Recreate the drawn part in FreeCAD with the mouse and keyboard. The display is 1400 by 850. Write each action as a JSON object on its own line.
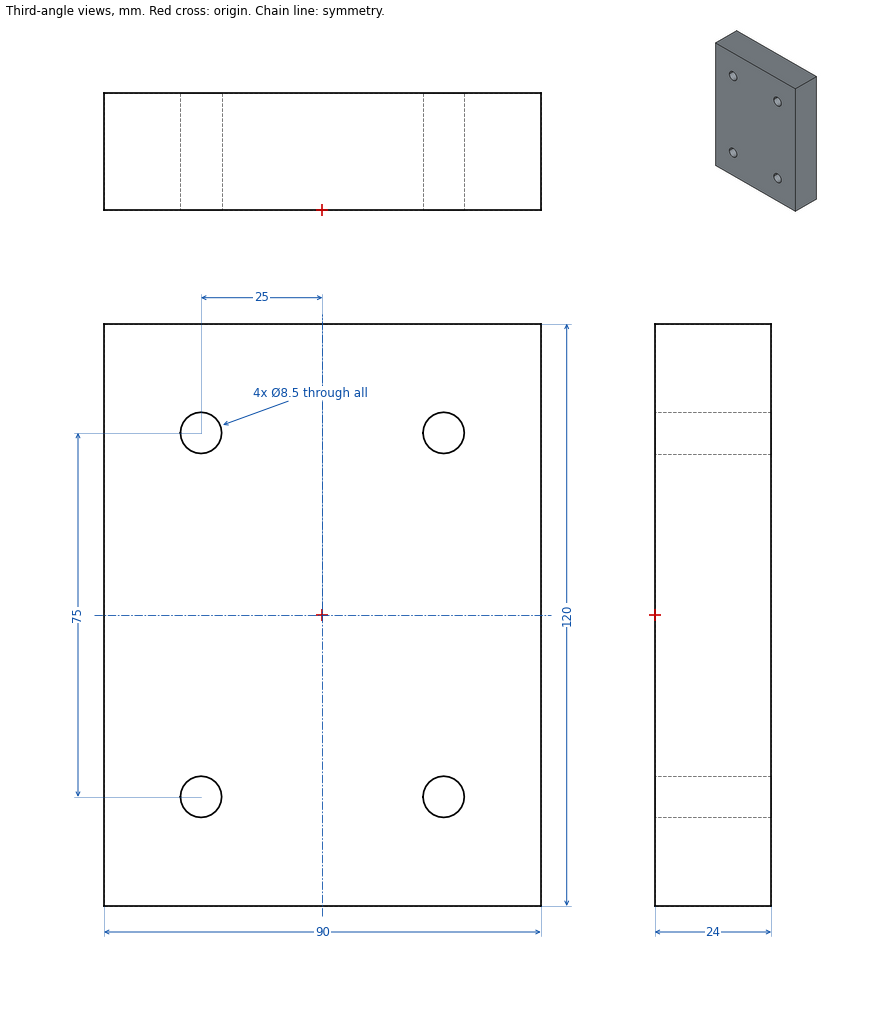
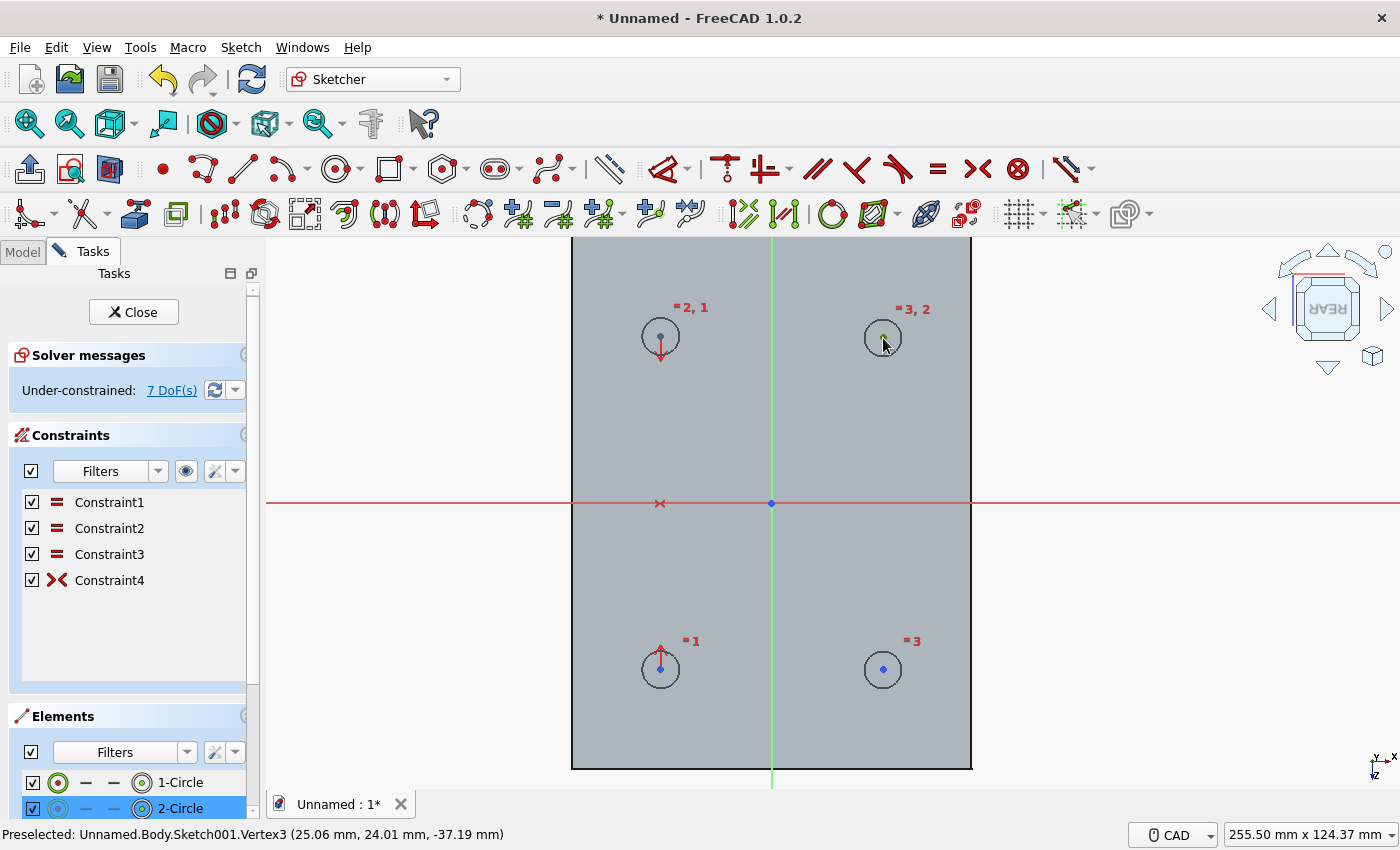
{"action": "left_click", "coordinate": [772, 726]}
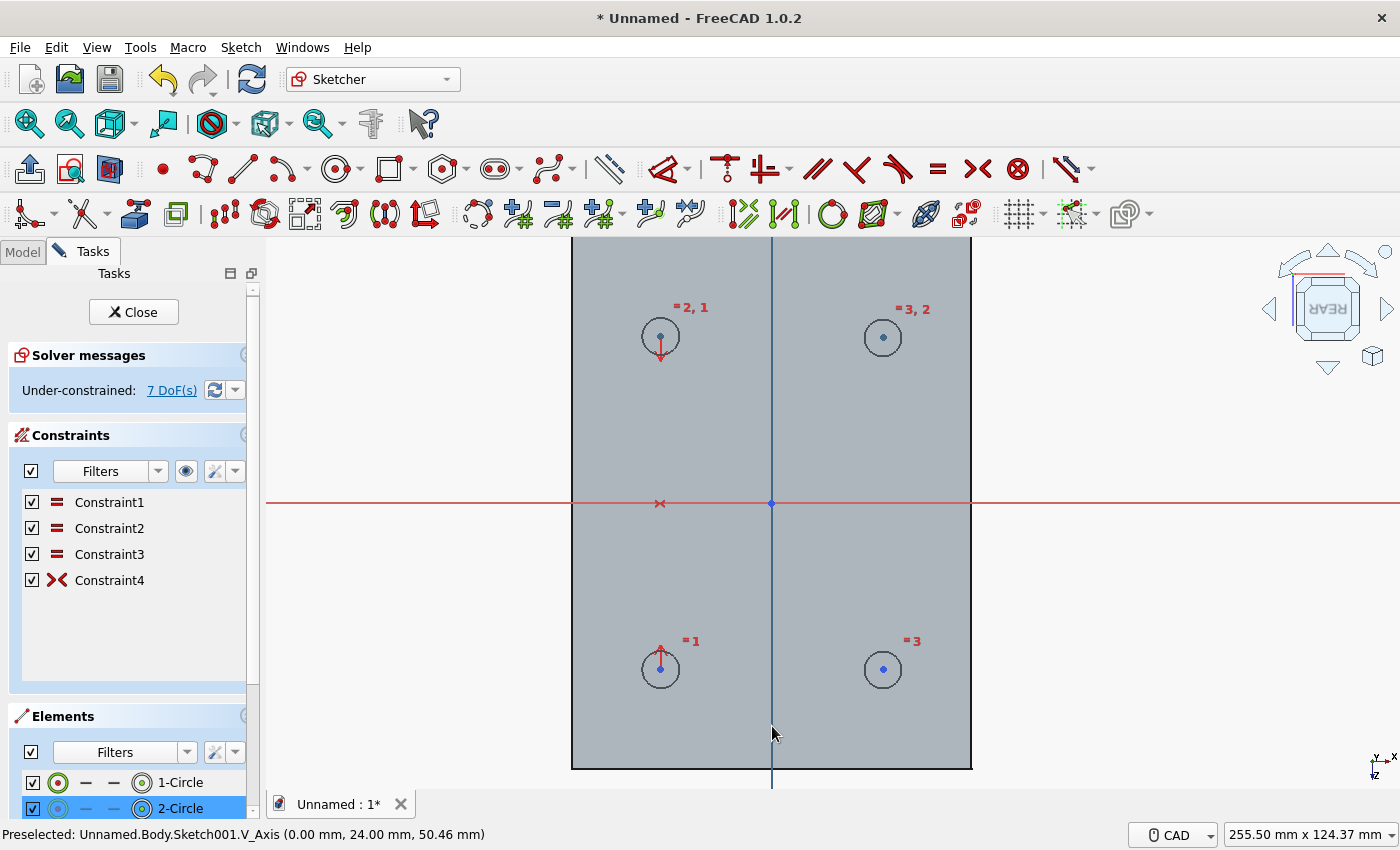
{"action": "key", "text": "s"}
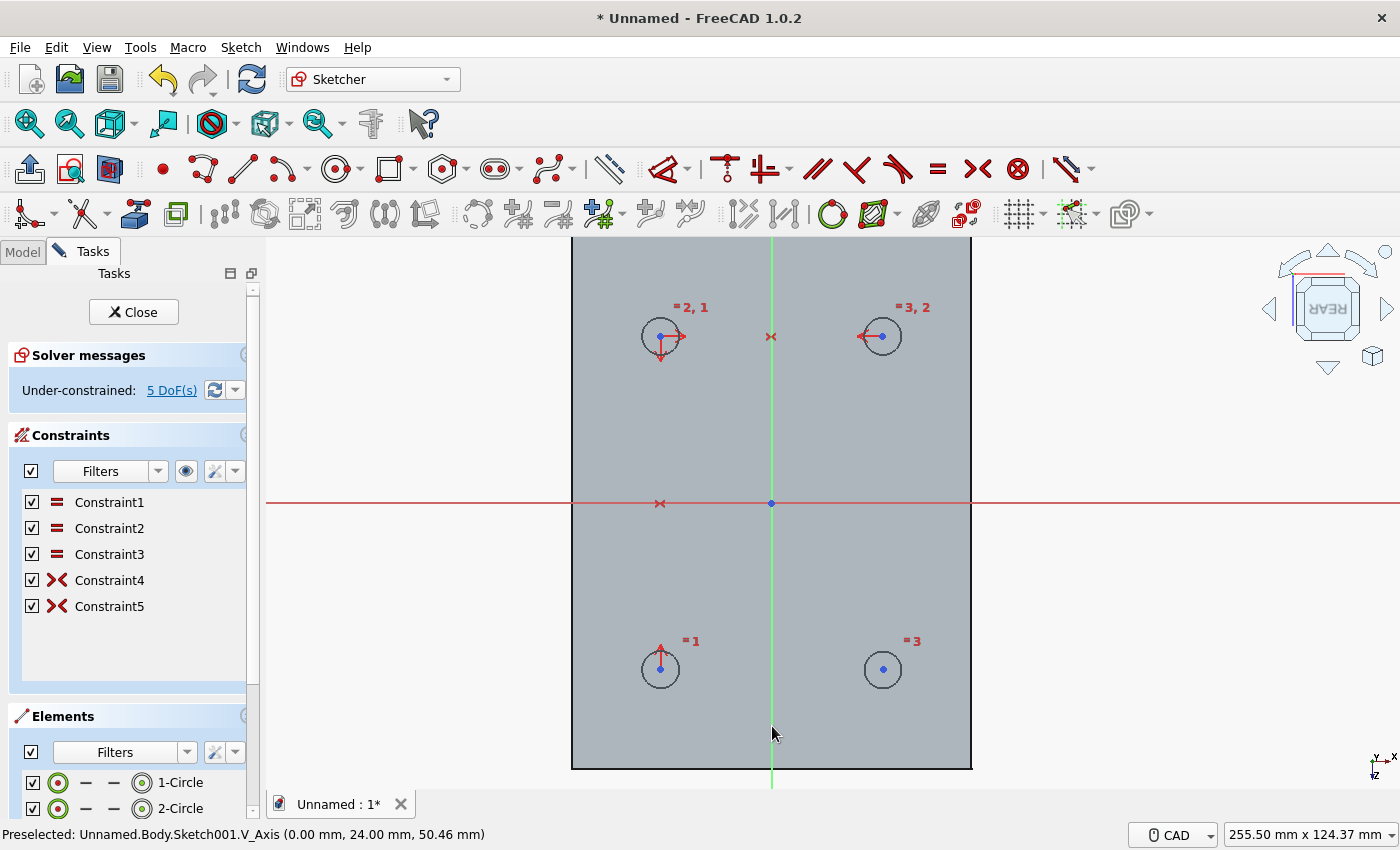
{"action": "left_click", "coordinate": [661, 670]}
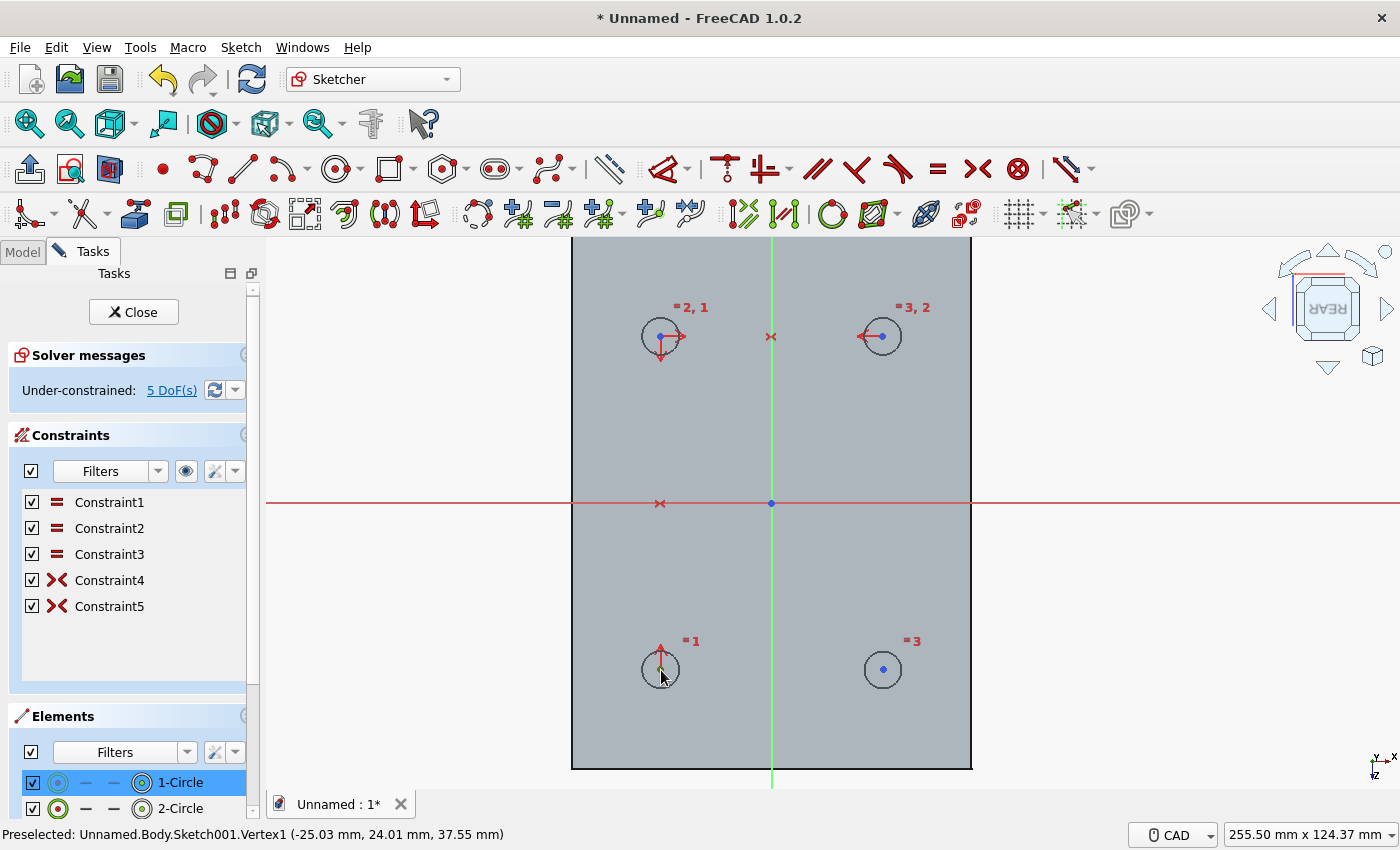
{"action": "left_click", "coordinate": [883, 670]}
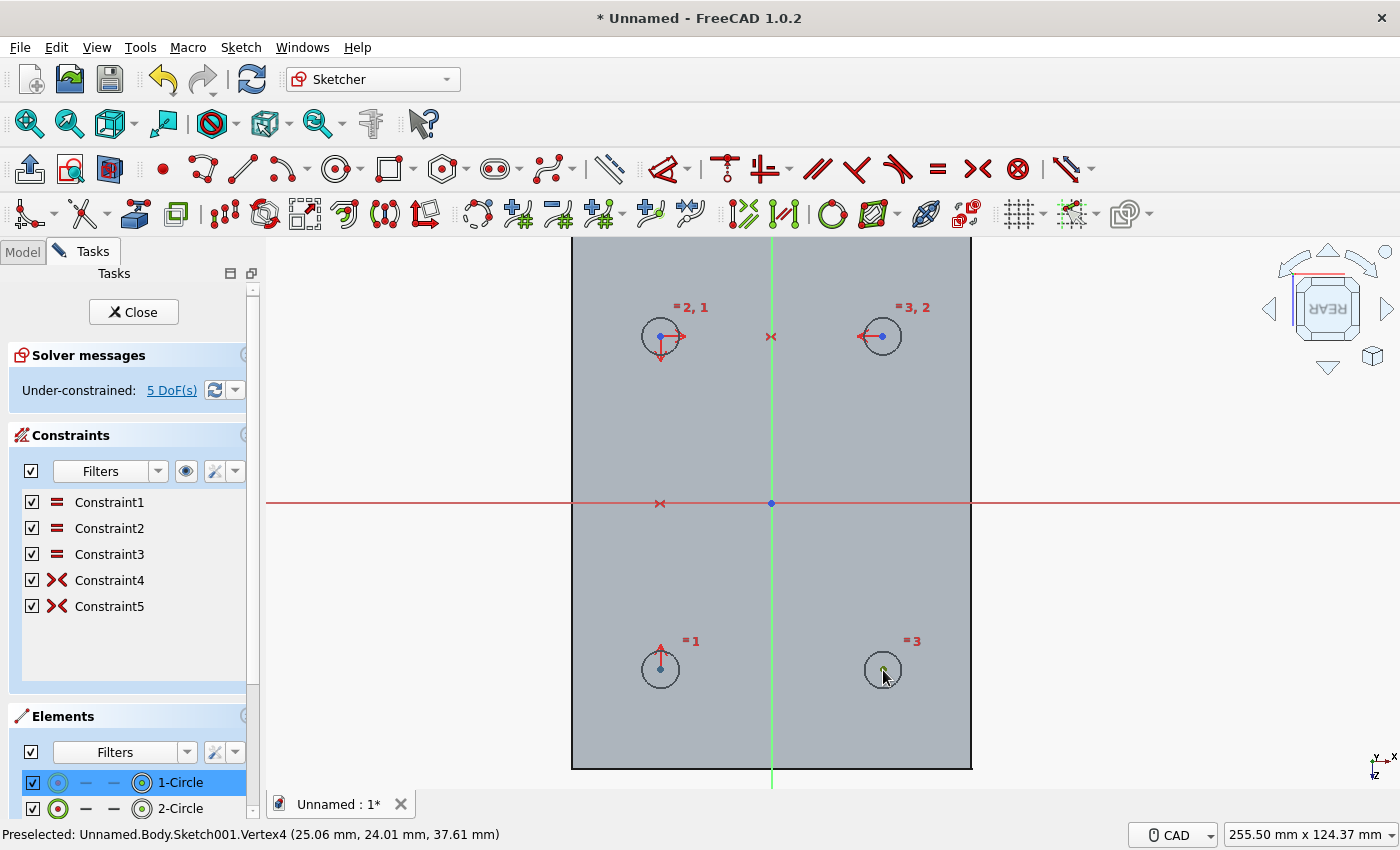
{"action": "left_click", "coordinate": [772, 726]}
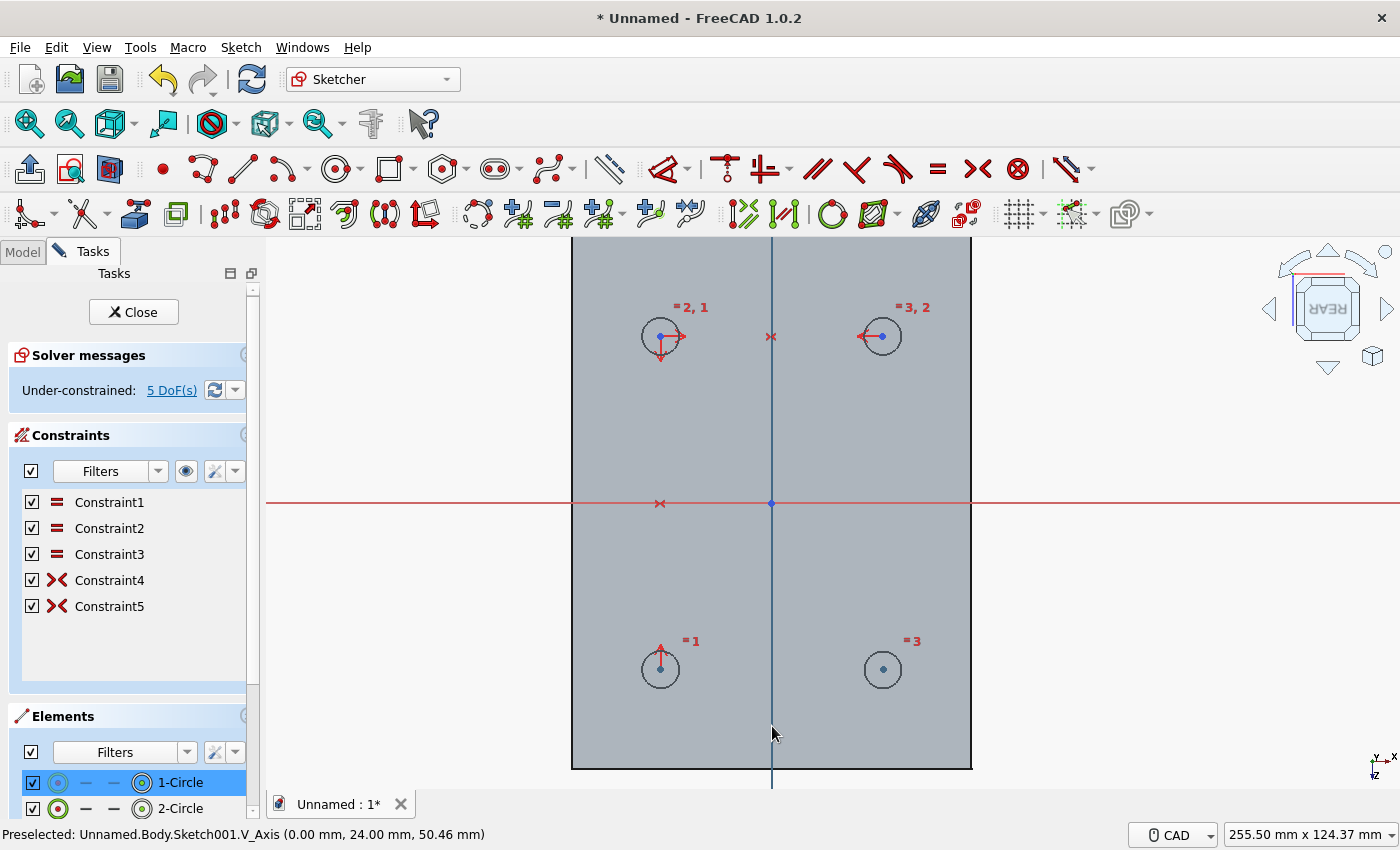
{"action": "key", "text": "s"}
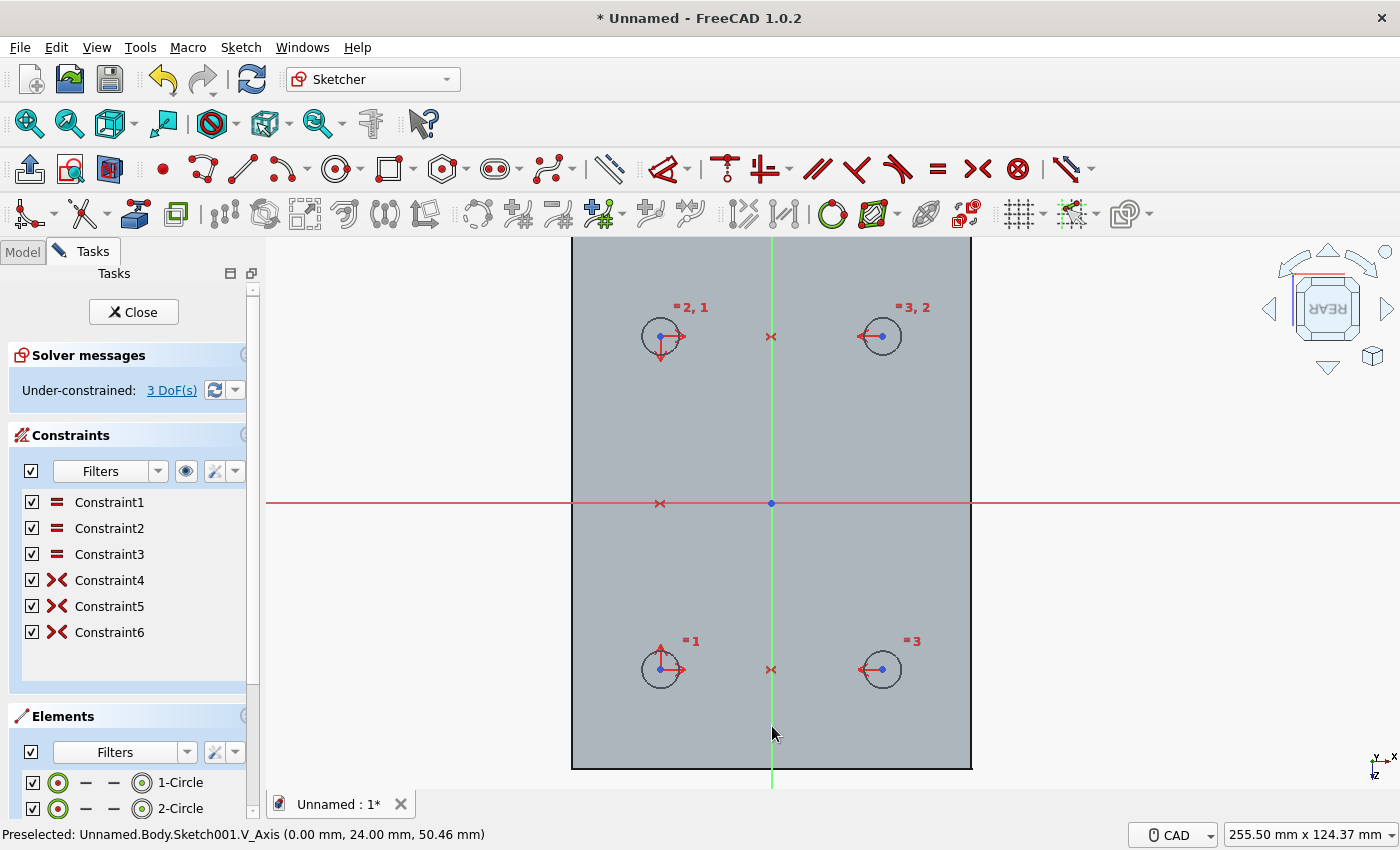
{"action": "left_click", "coordinate": [674, 657]}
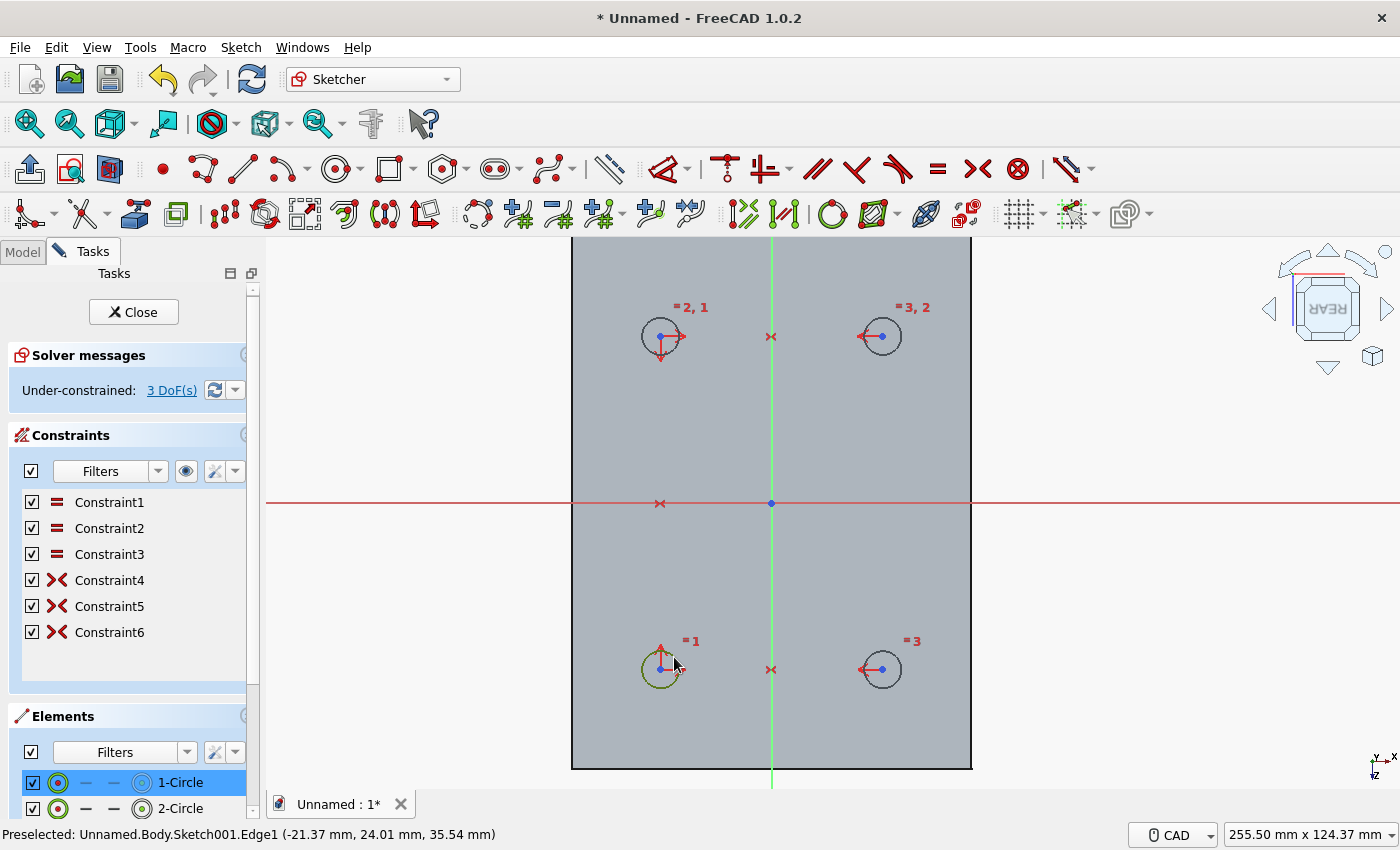
{"action": "key", "text": "k o"}